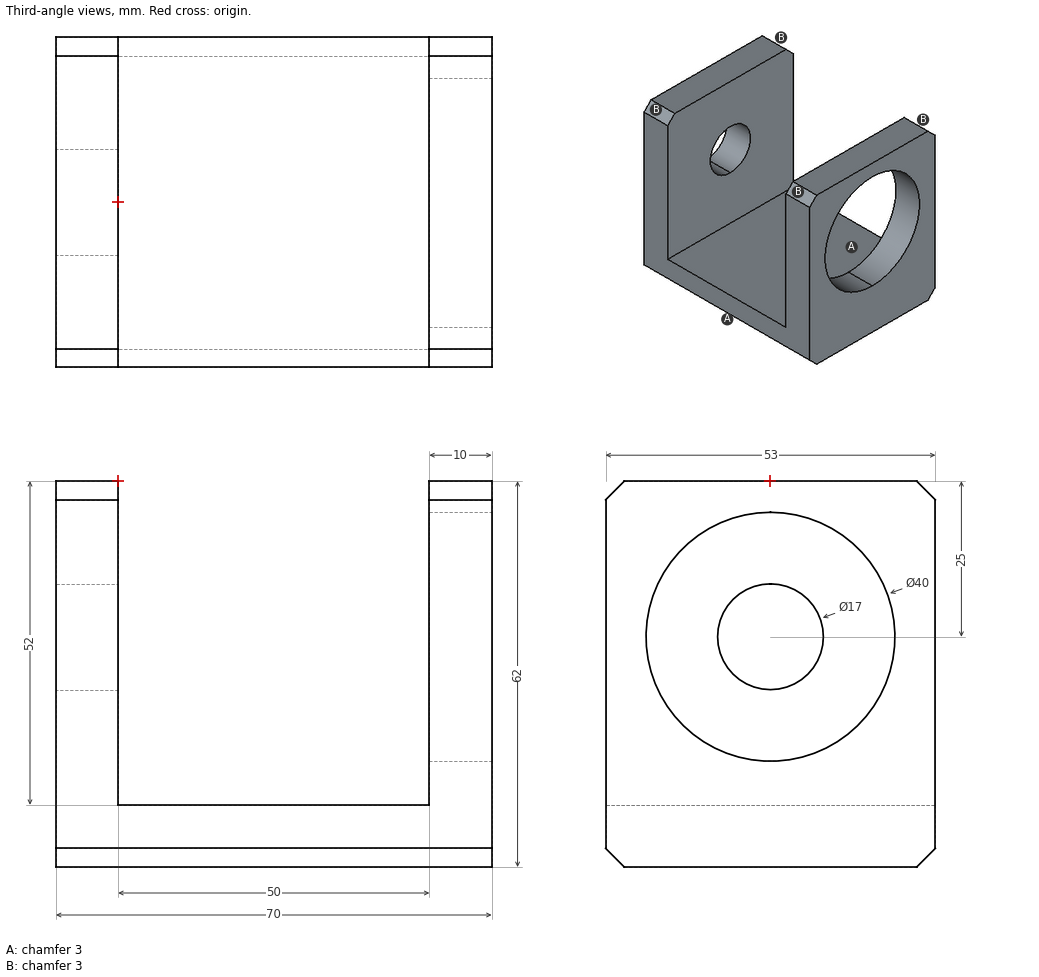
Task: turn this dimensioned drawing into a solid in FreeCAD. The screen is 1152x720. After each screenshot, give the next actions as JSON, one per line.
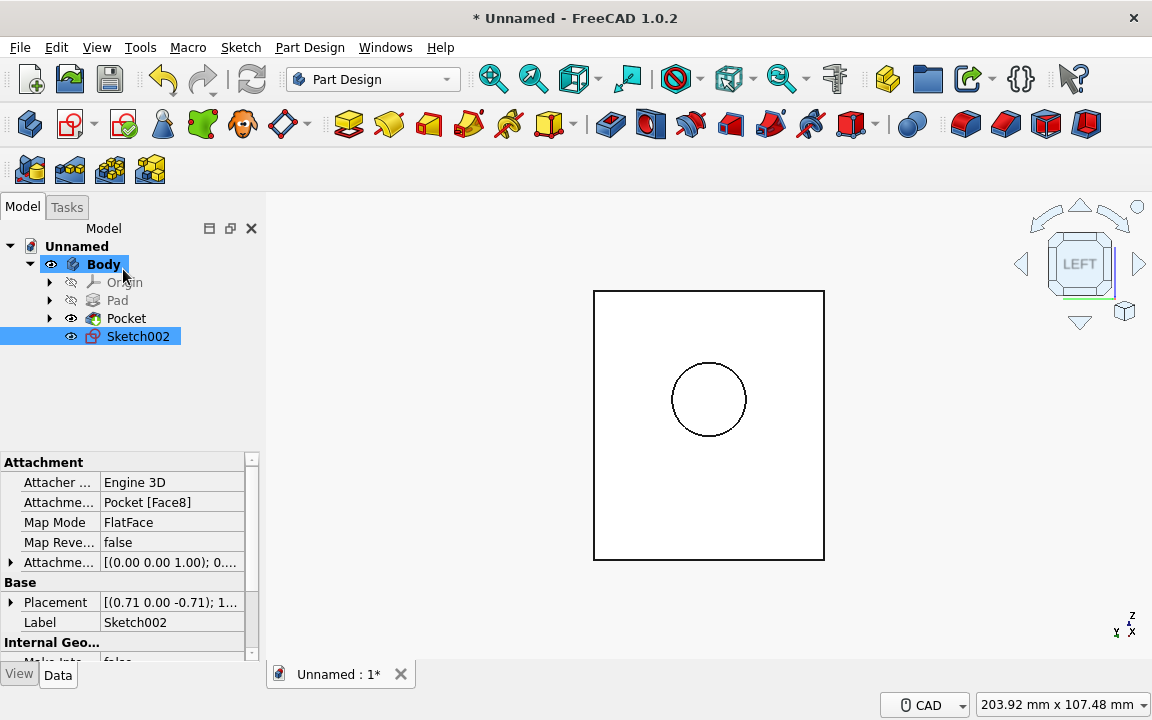
{"action": "left_click", "coordinate": [612, 124]}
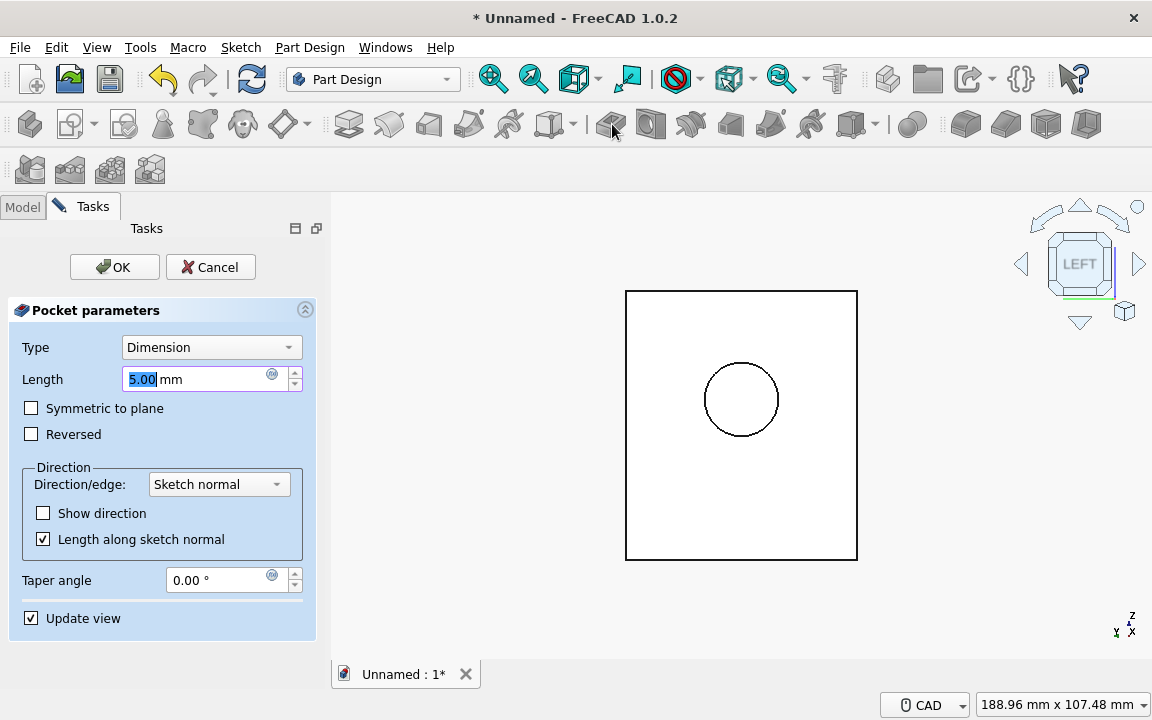
{"action": "left_click", "coordinate": [212, 348]}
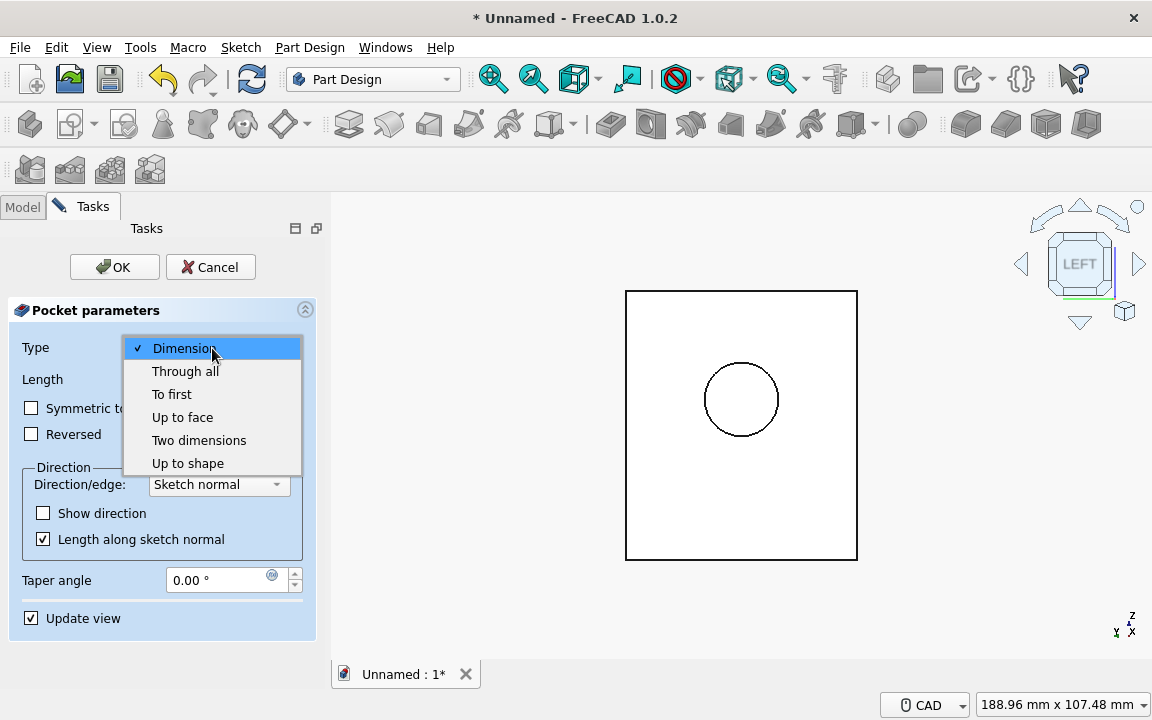
{"action": "left_click", "coordinate": [212, 394]}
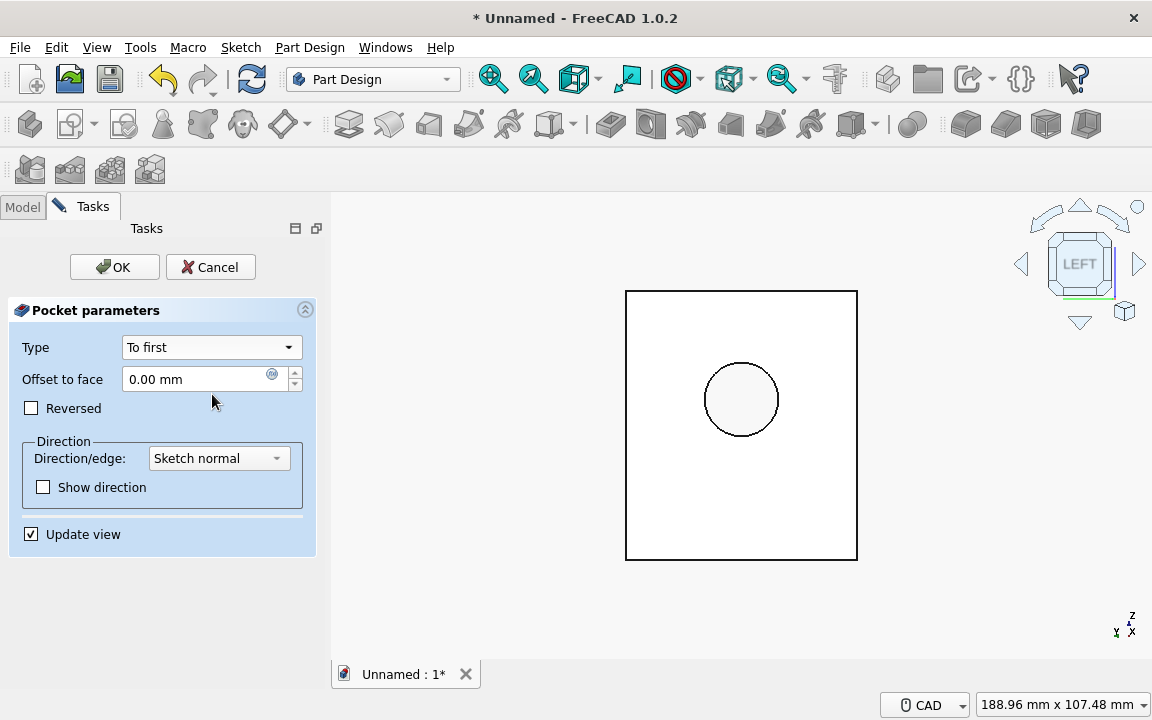
{"action": "left_click", "coordinate": [115, 267]}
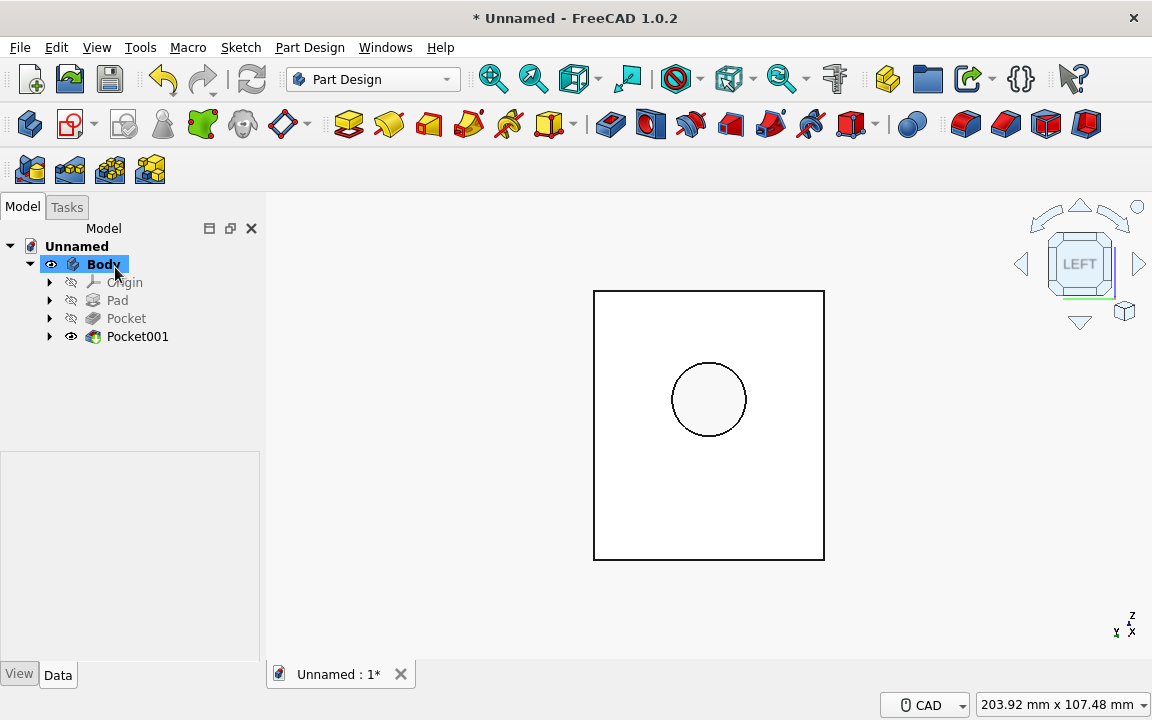
{"action": "key", "text": "0"}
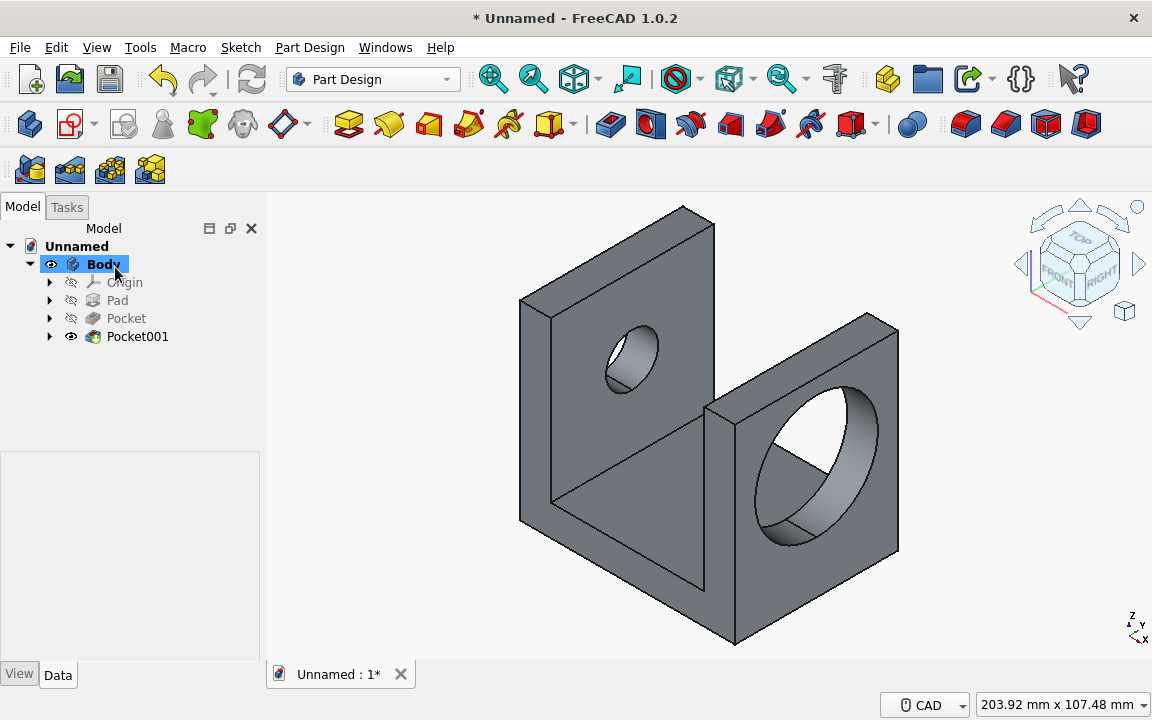
{"action": "key", "text": "2"}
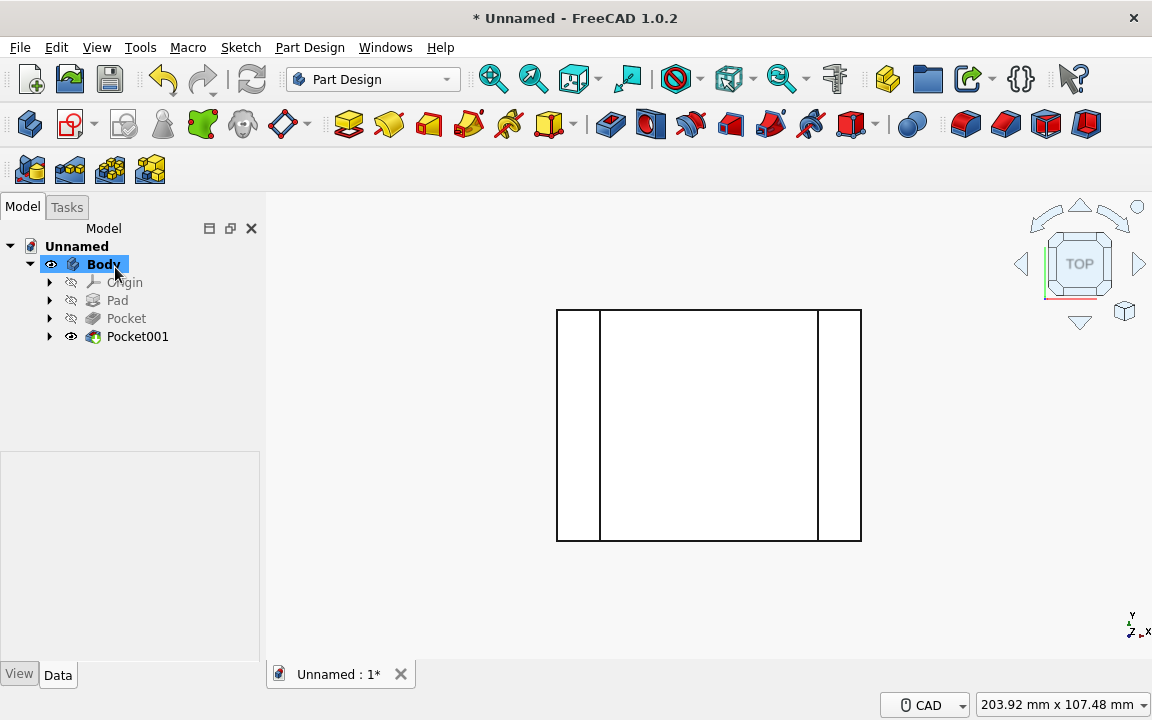
{"action": "key", "text": "1"}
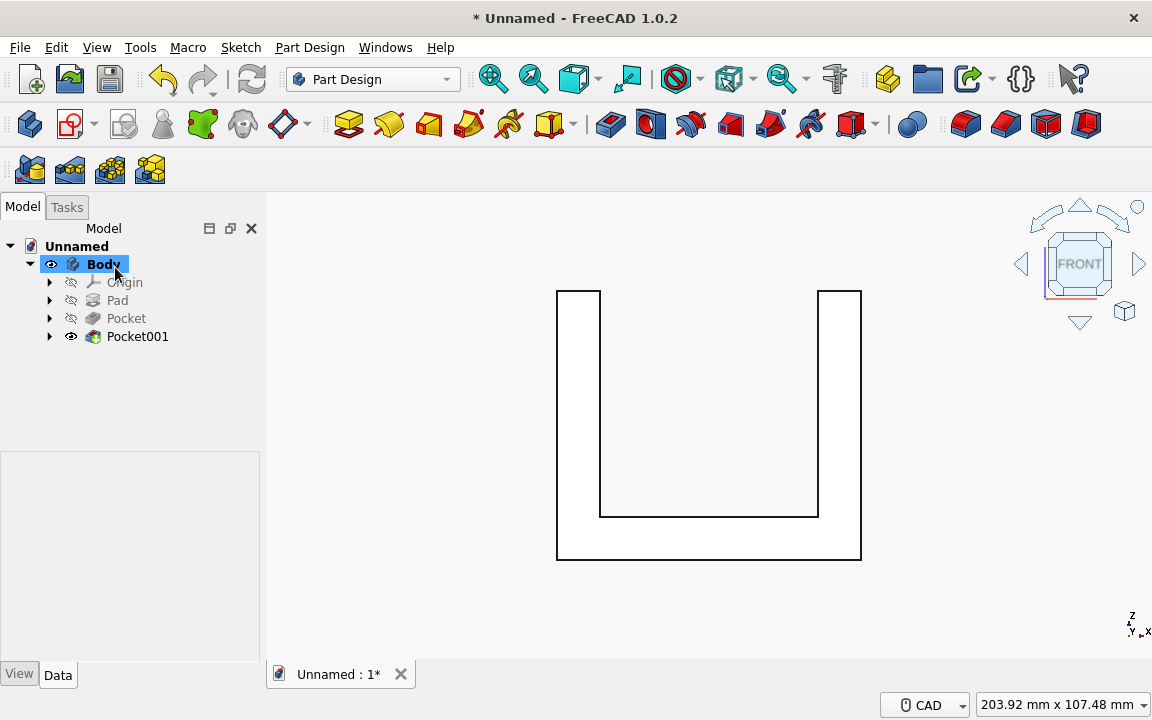
{"action": "key", "text": "3"}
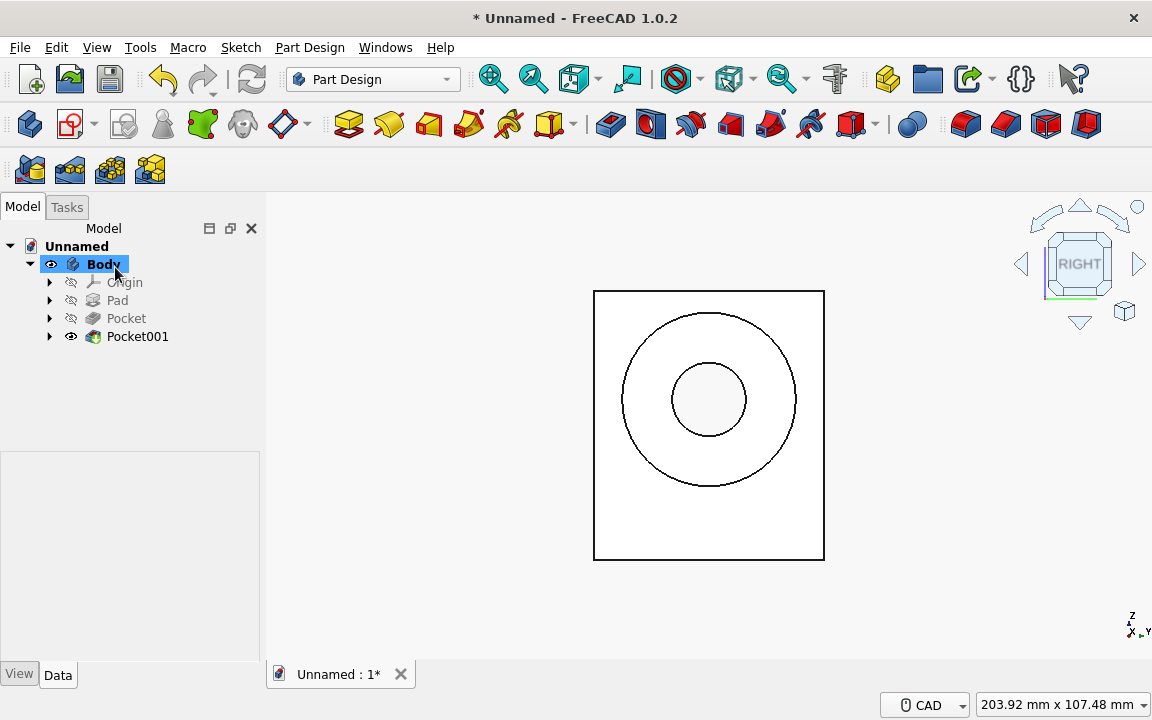
{"action": "key", "text": "5"}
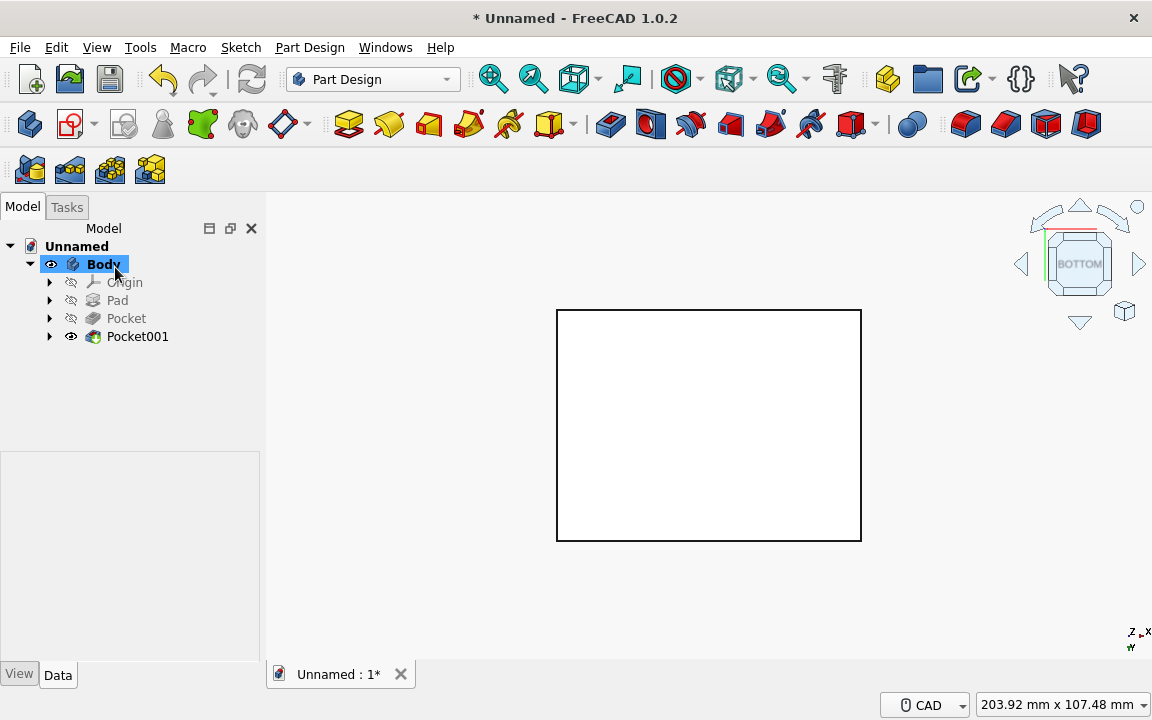
{"action": "left_click", "coordinate": [709, 309]}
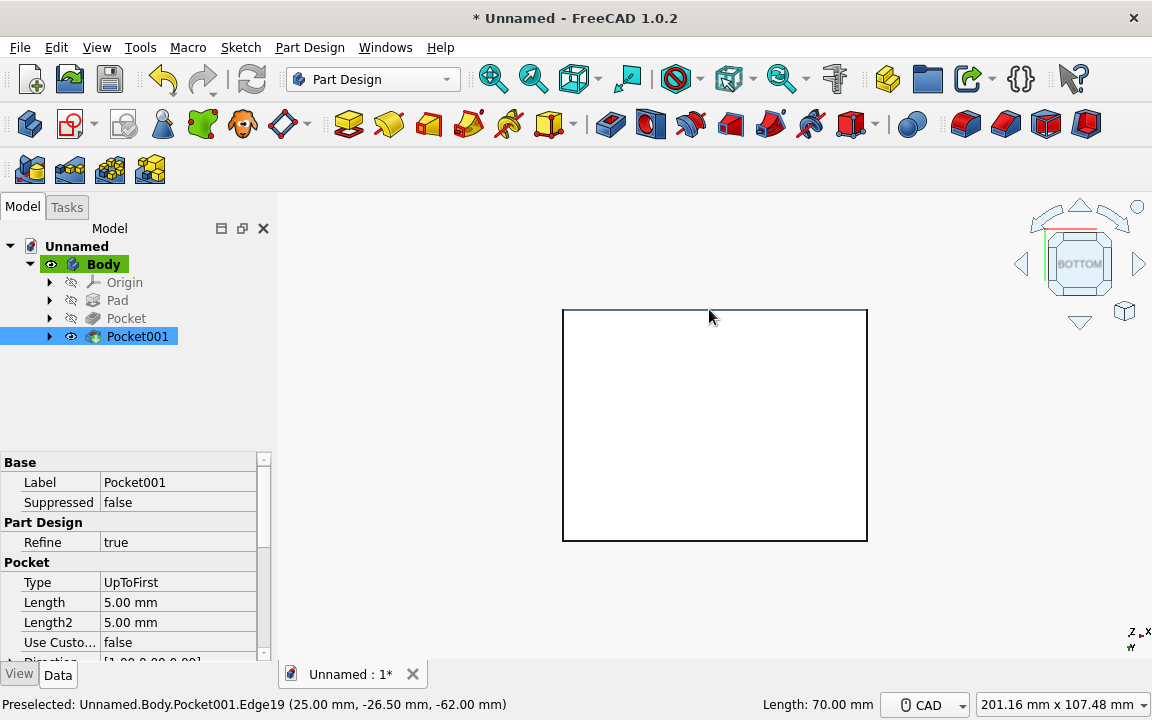
{"action": "key", "text": "4"}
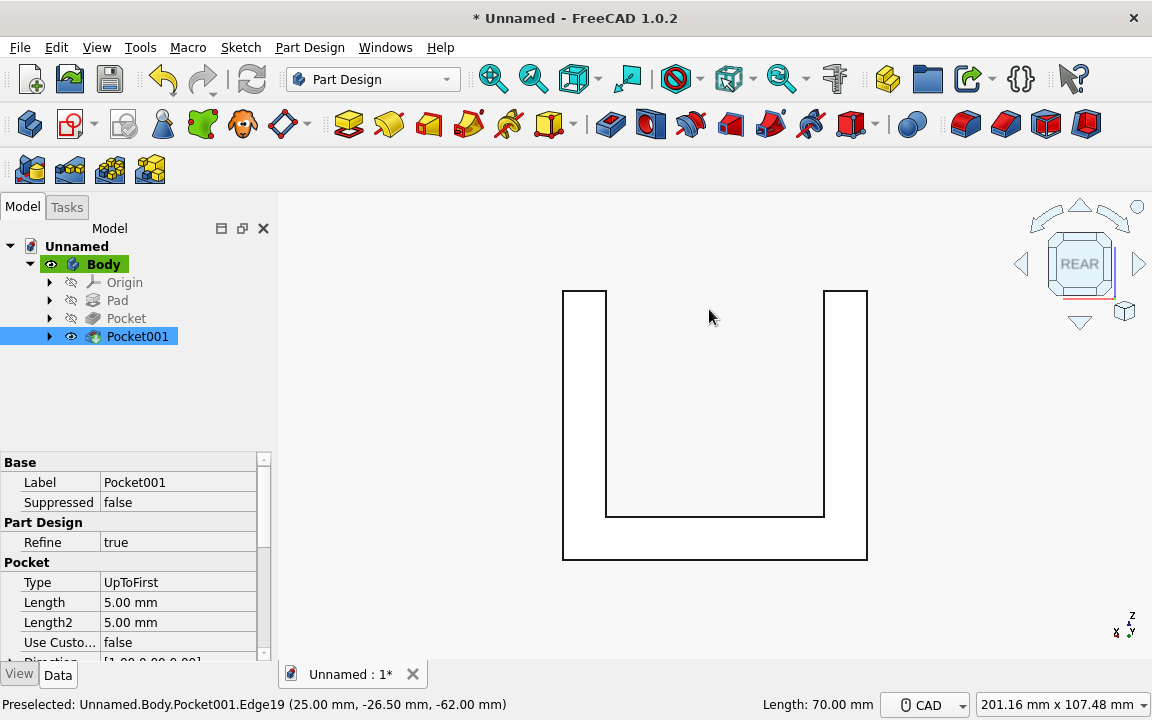
{"action": "left_click", "coordinate": [715, 559], "text": "ctrl"}